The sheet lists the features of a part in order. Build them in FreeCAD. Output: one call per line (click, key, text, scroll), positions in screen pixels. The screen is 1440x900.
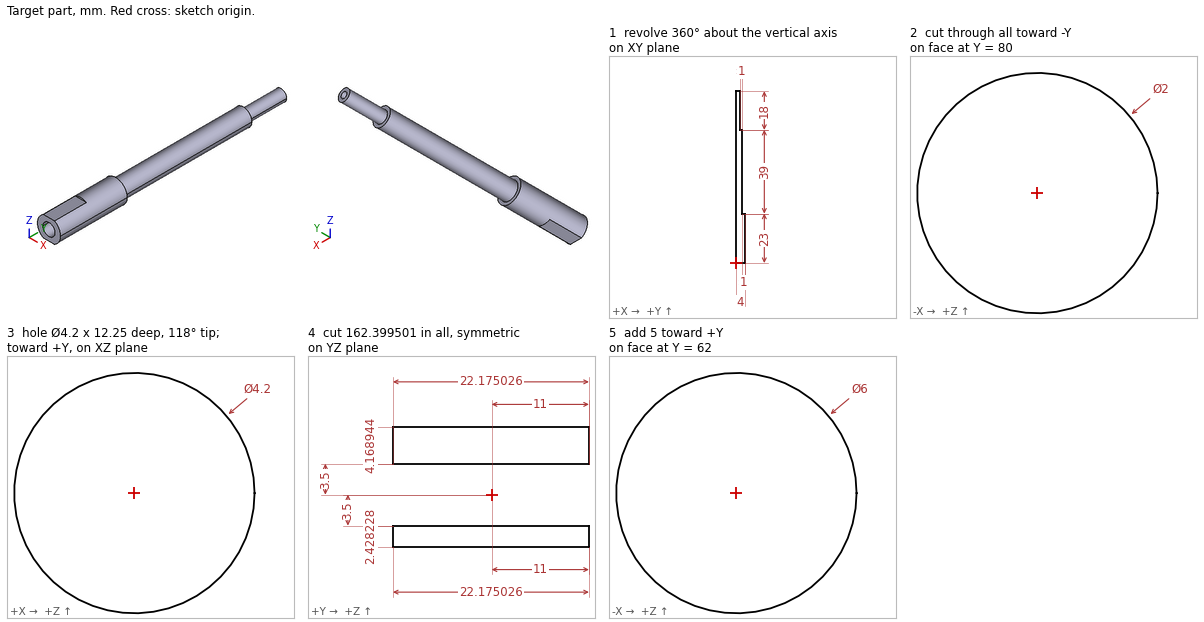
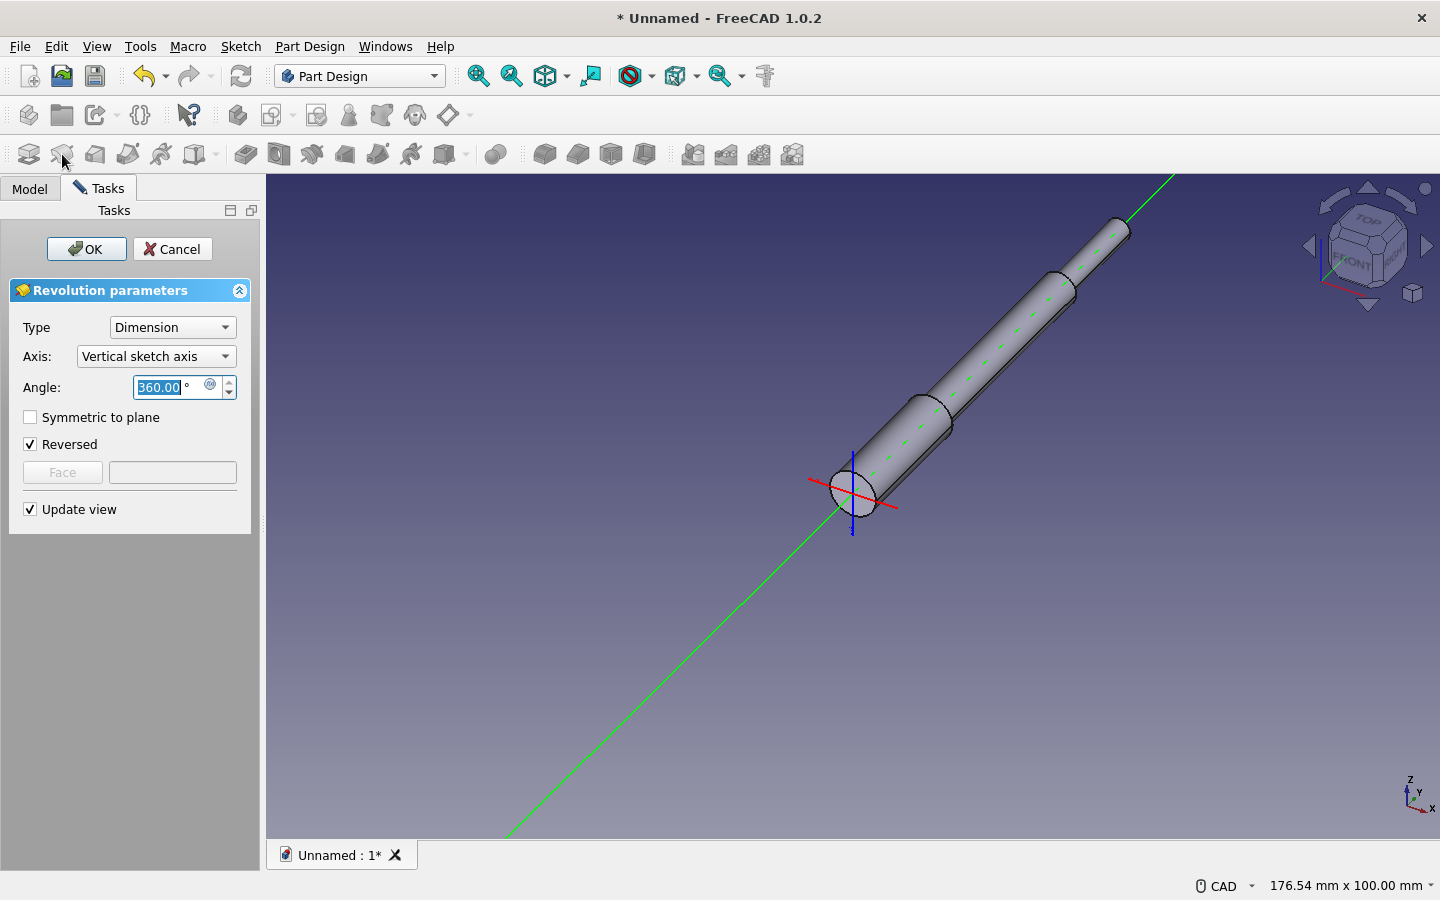
click(87, 249)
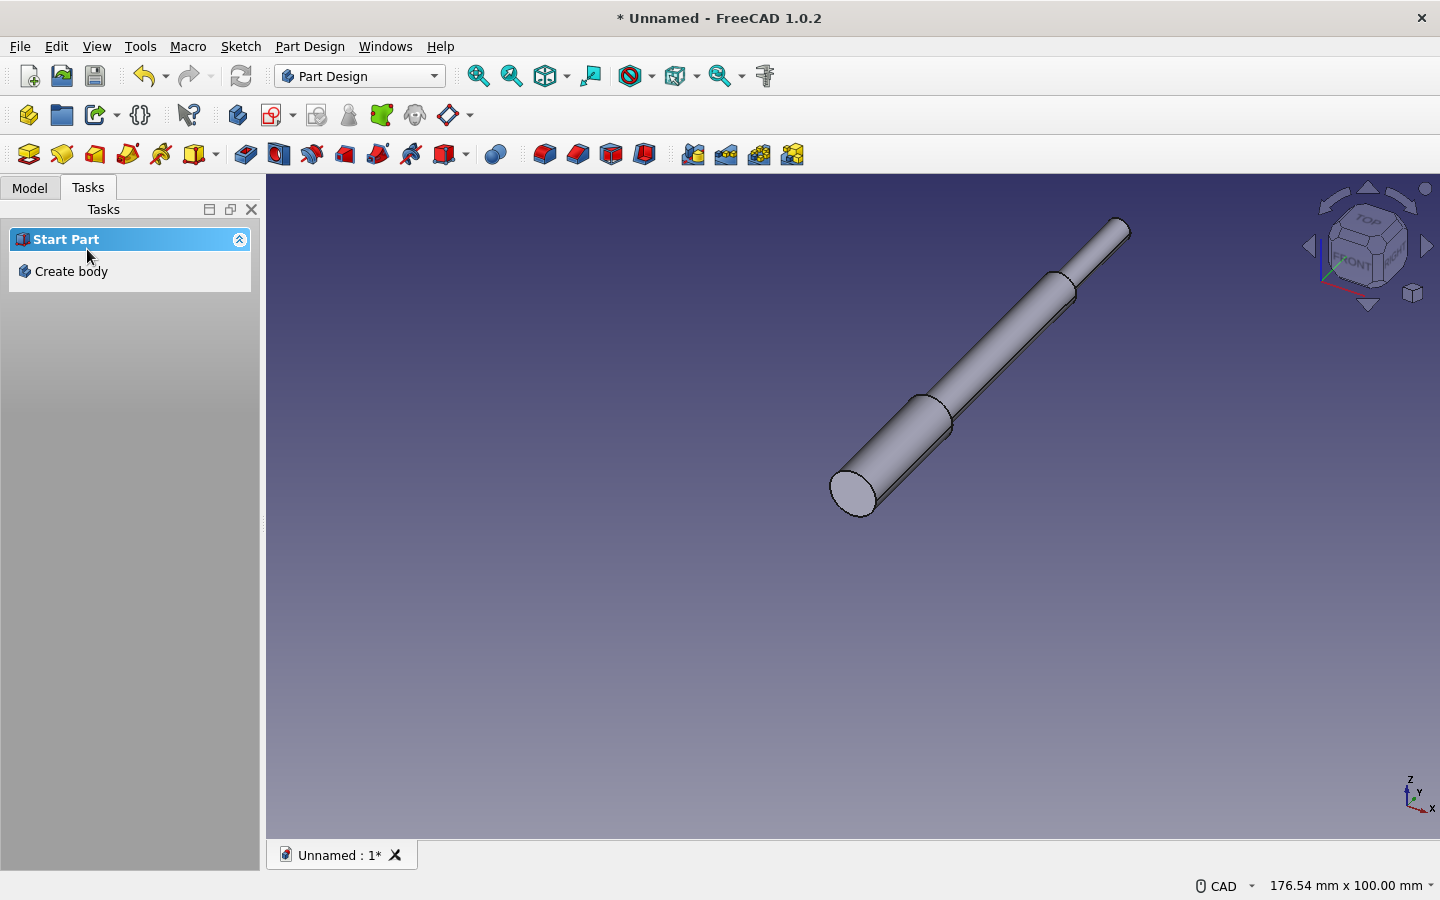
key(4)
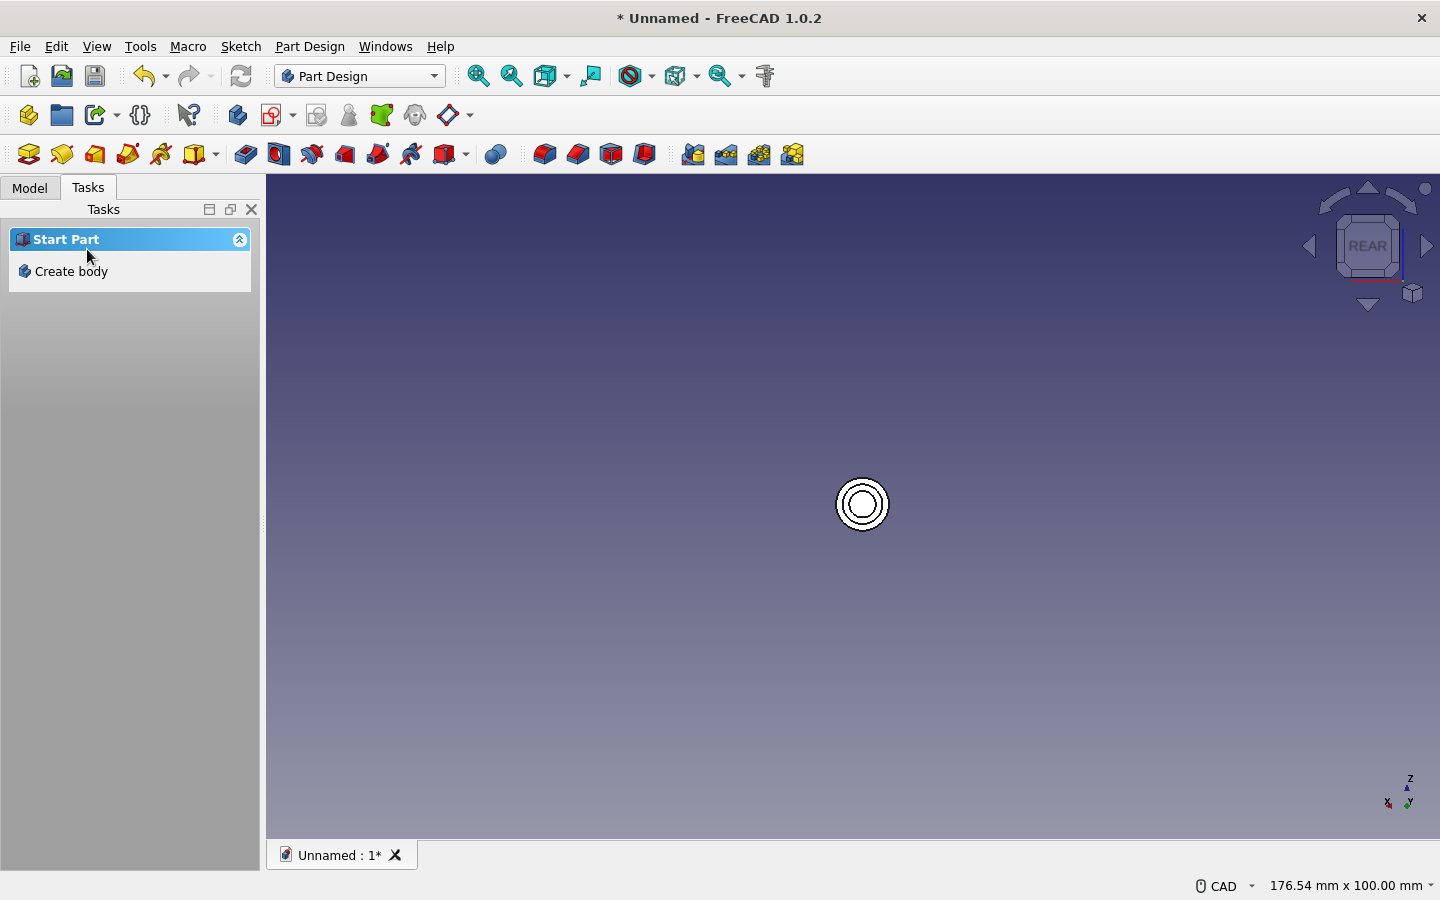
key(v)
key(f)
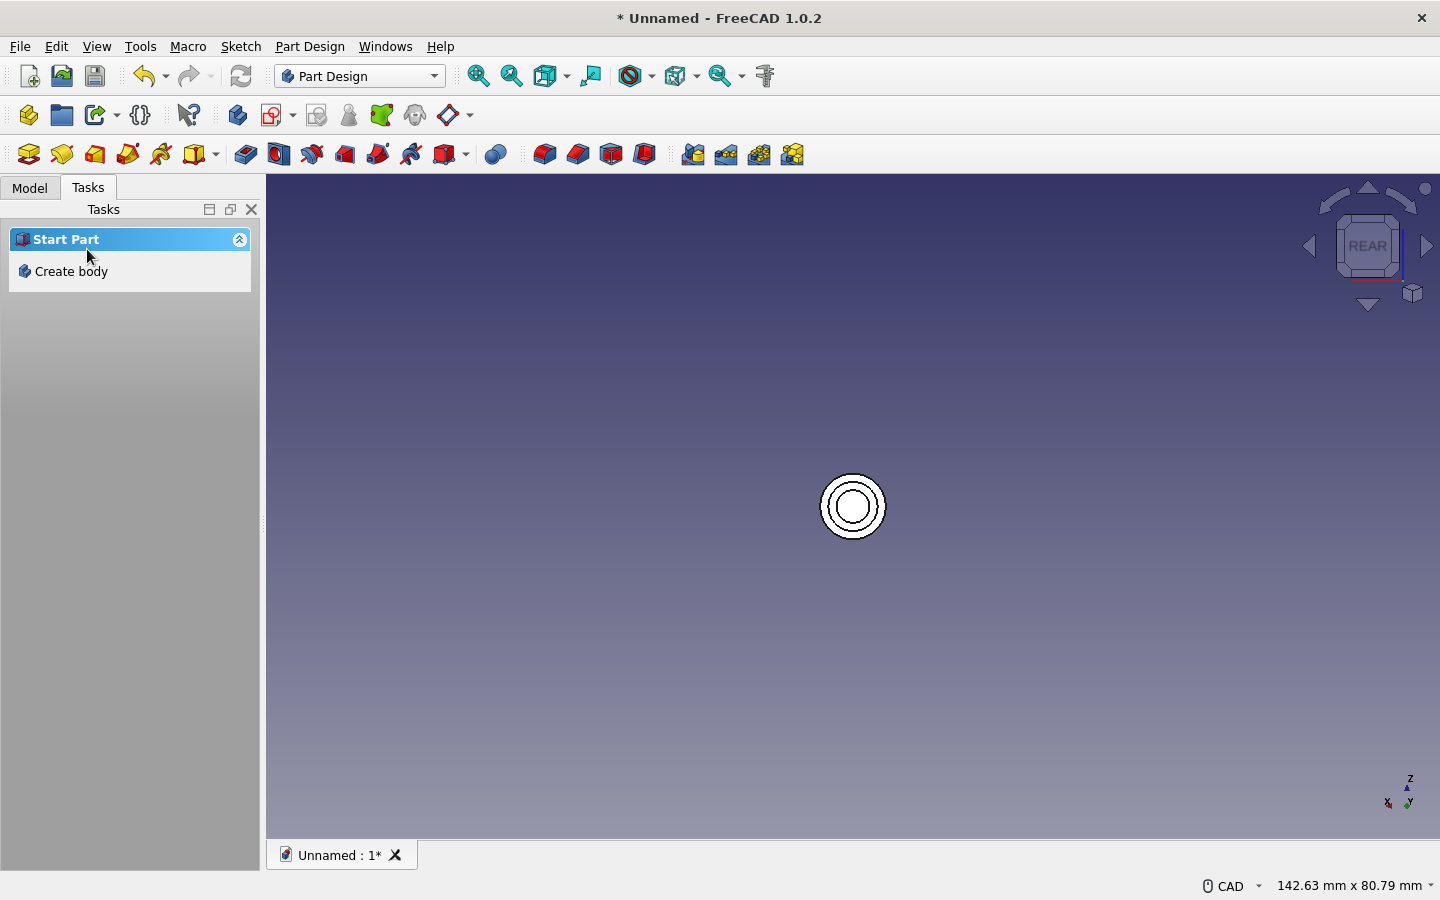
click(853, 506)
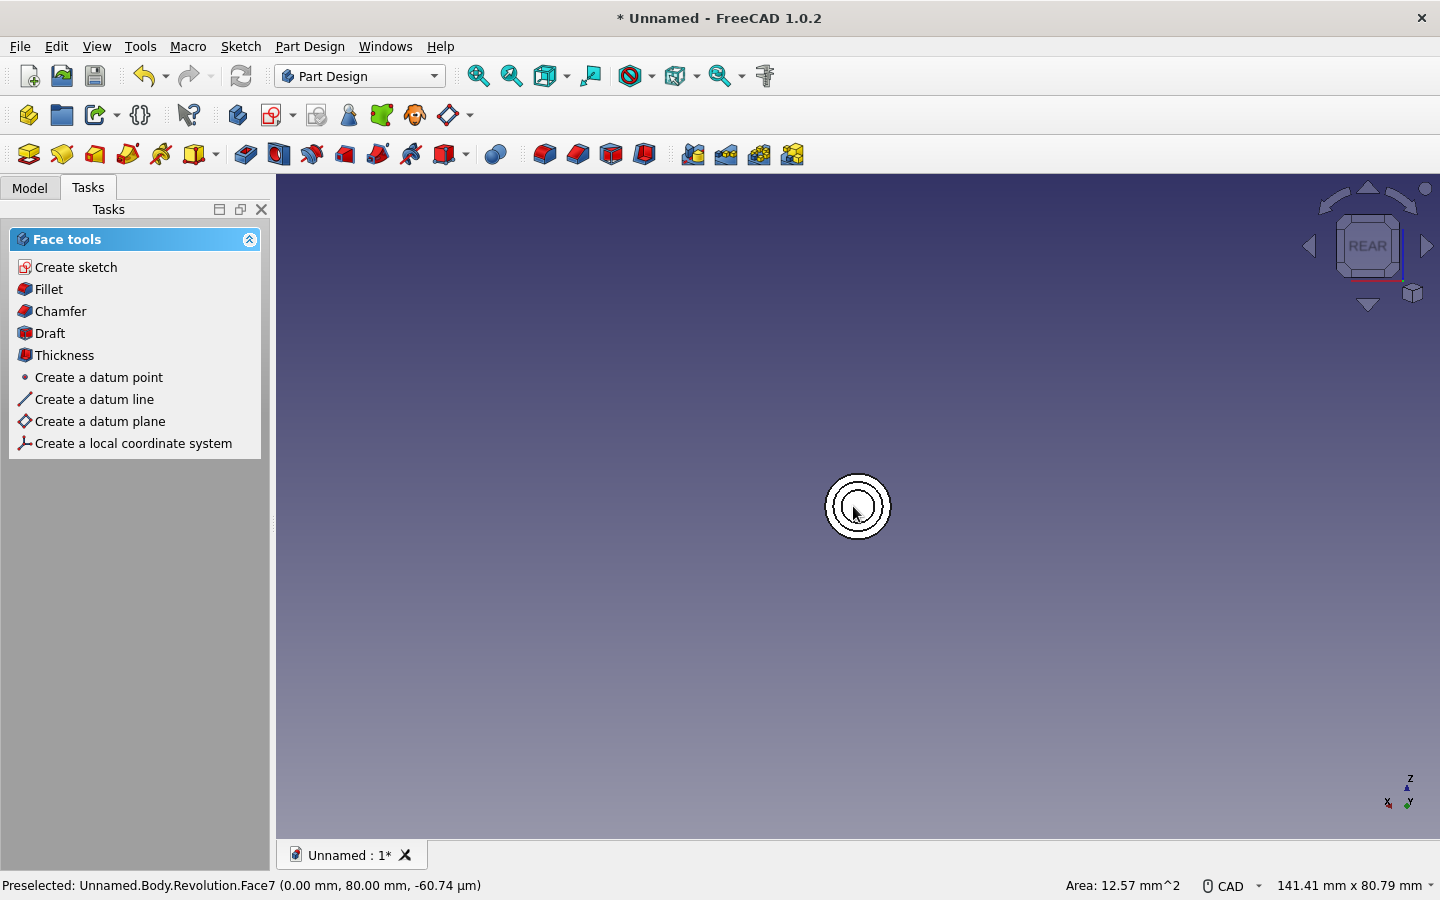
click(270, 116)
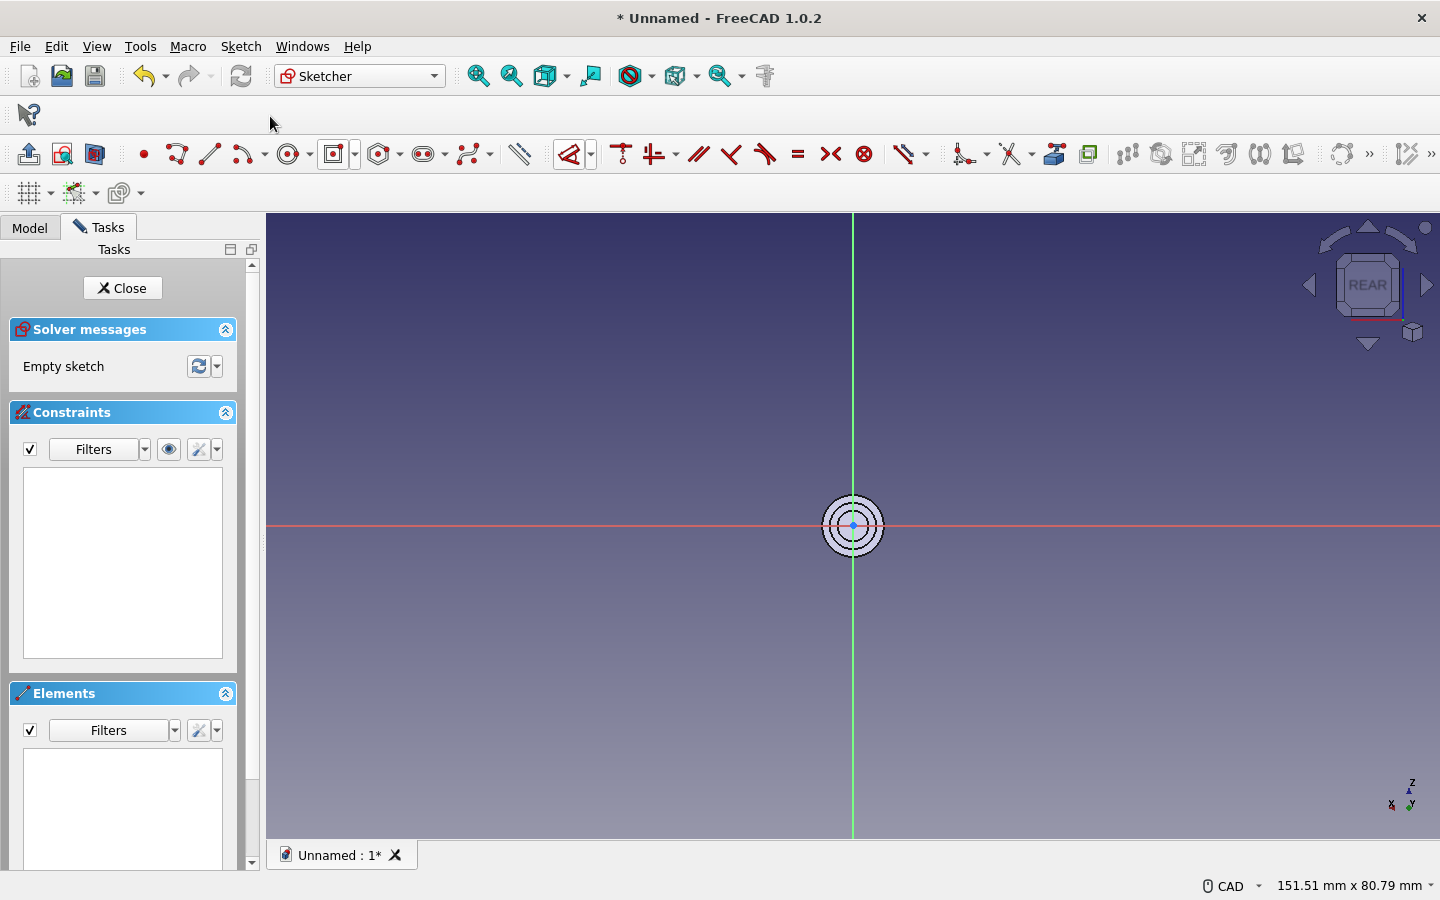
scroll(857, 526, up, 15)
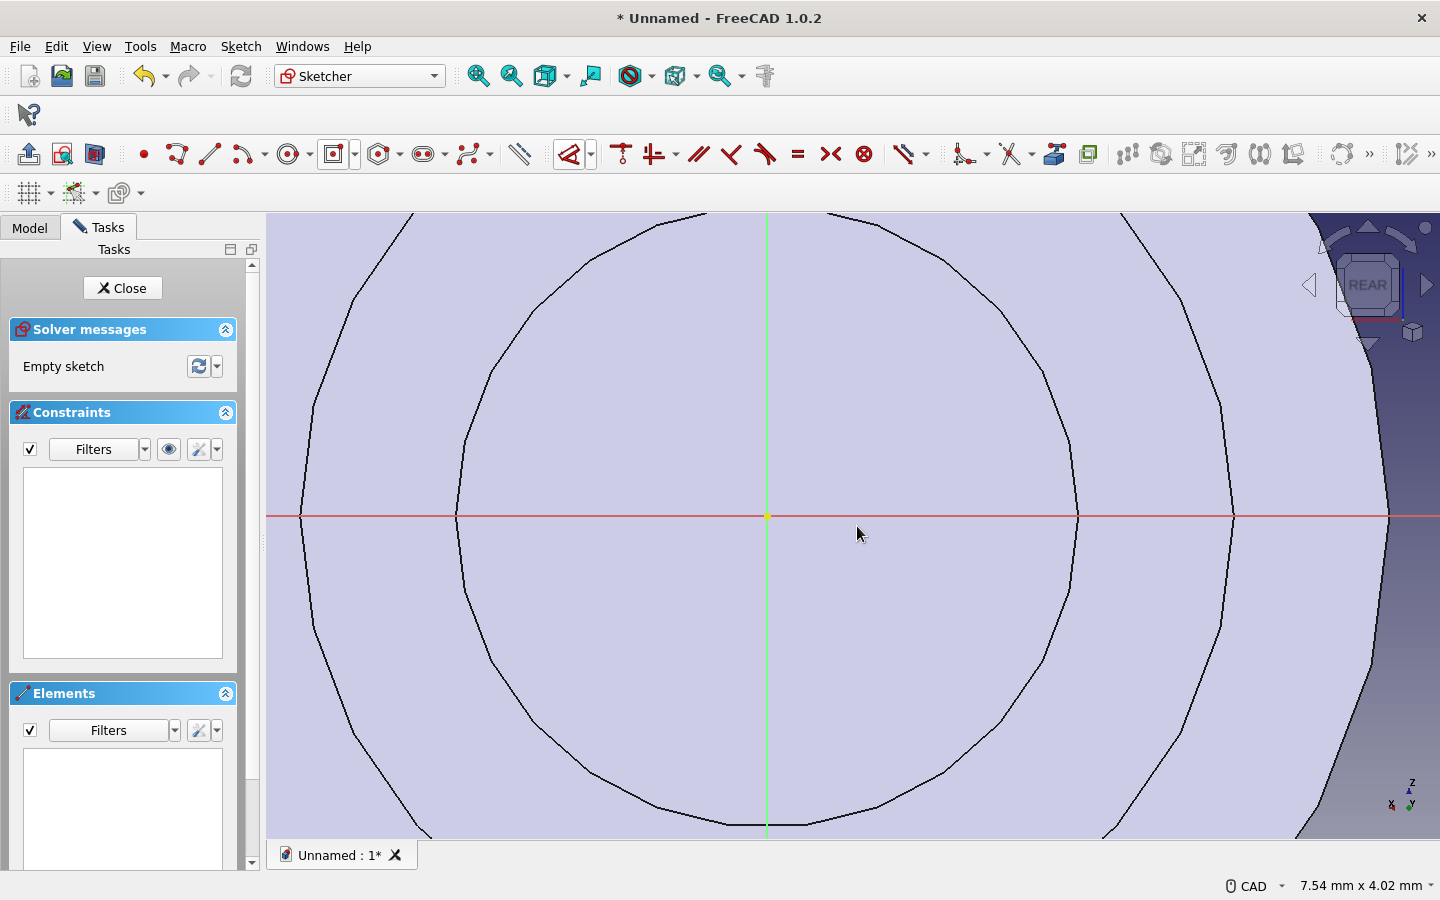
key(g)
key(c)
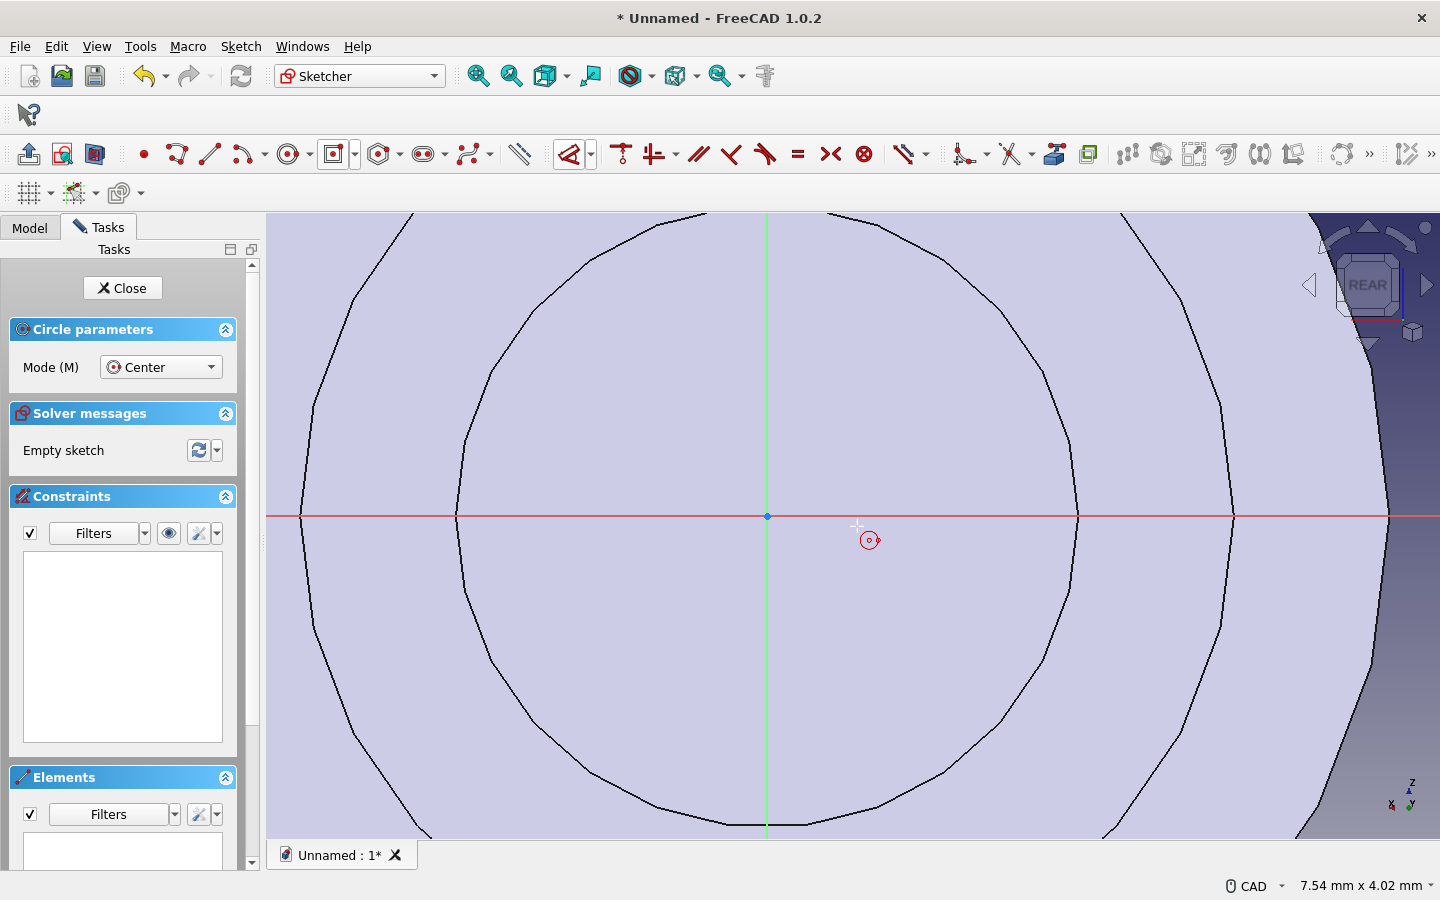
click(767, 516)
click(877, 406)
key(Escape)